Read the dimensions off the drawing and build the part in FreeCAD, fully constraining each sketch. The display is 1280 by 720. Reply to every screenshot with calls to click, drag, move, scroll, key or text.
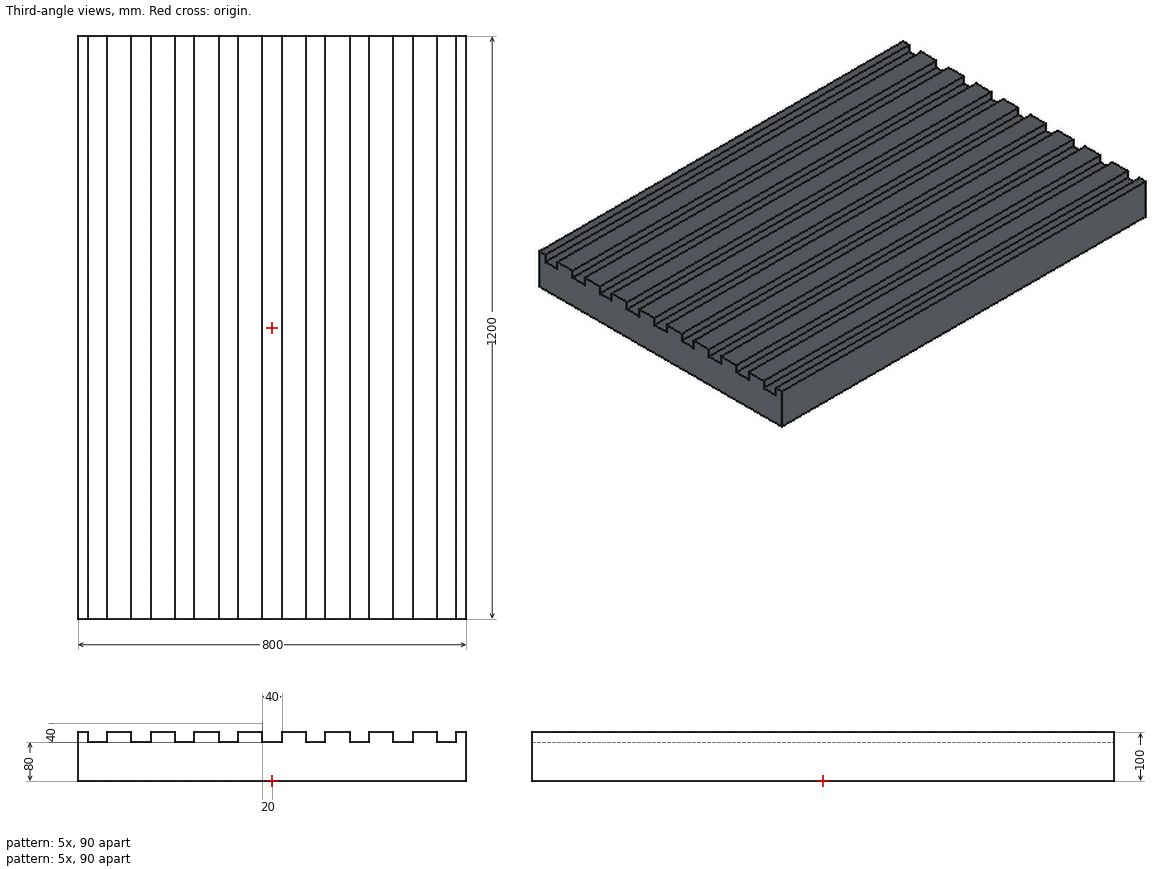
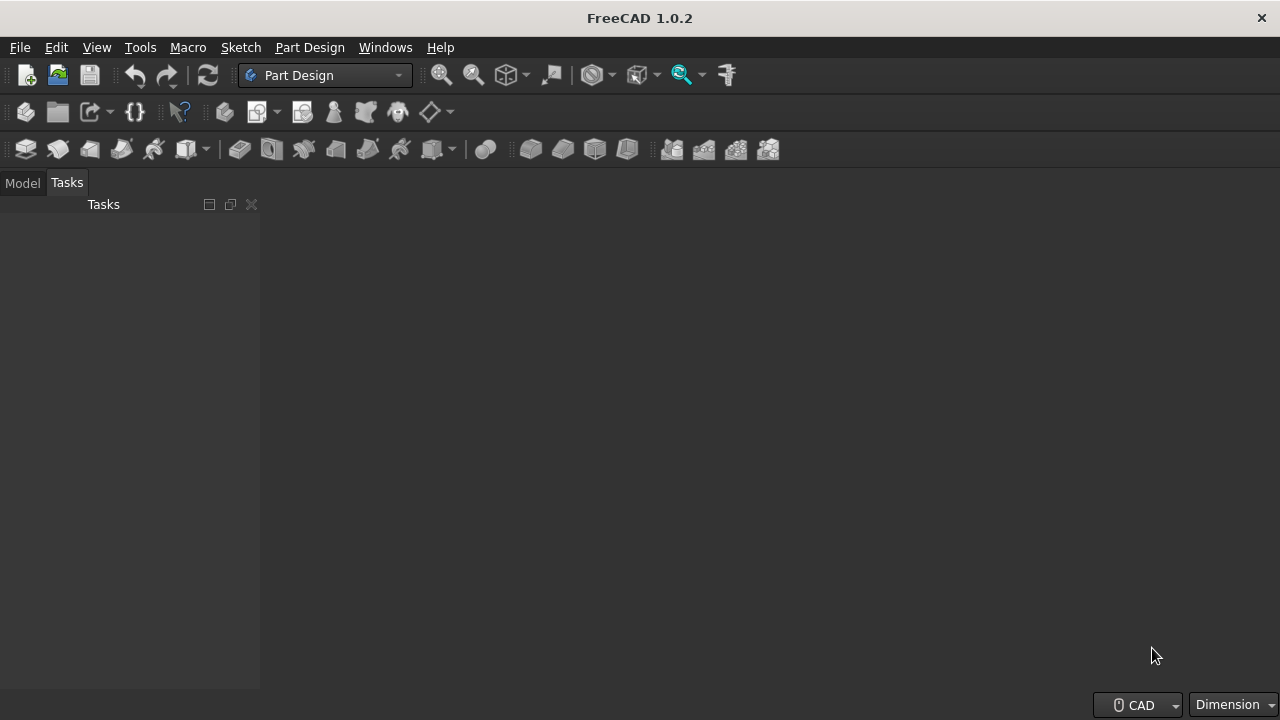
key(ctrl+n)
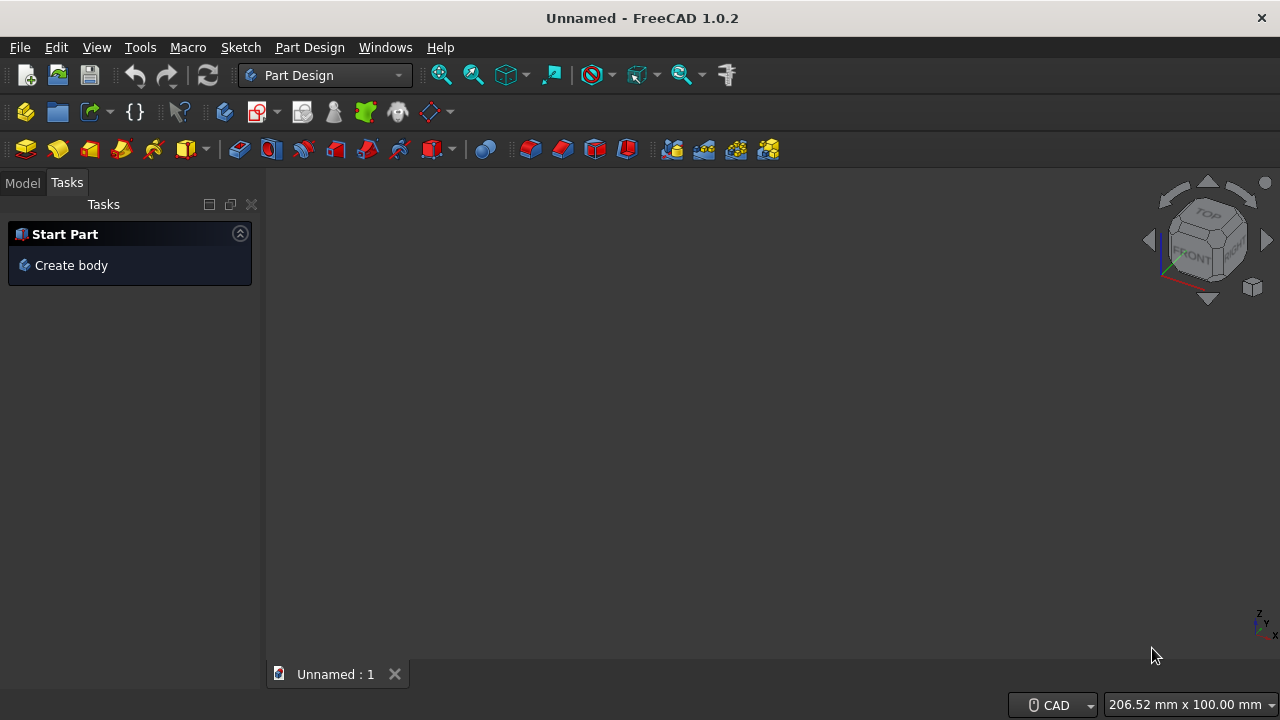
click(258, 112)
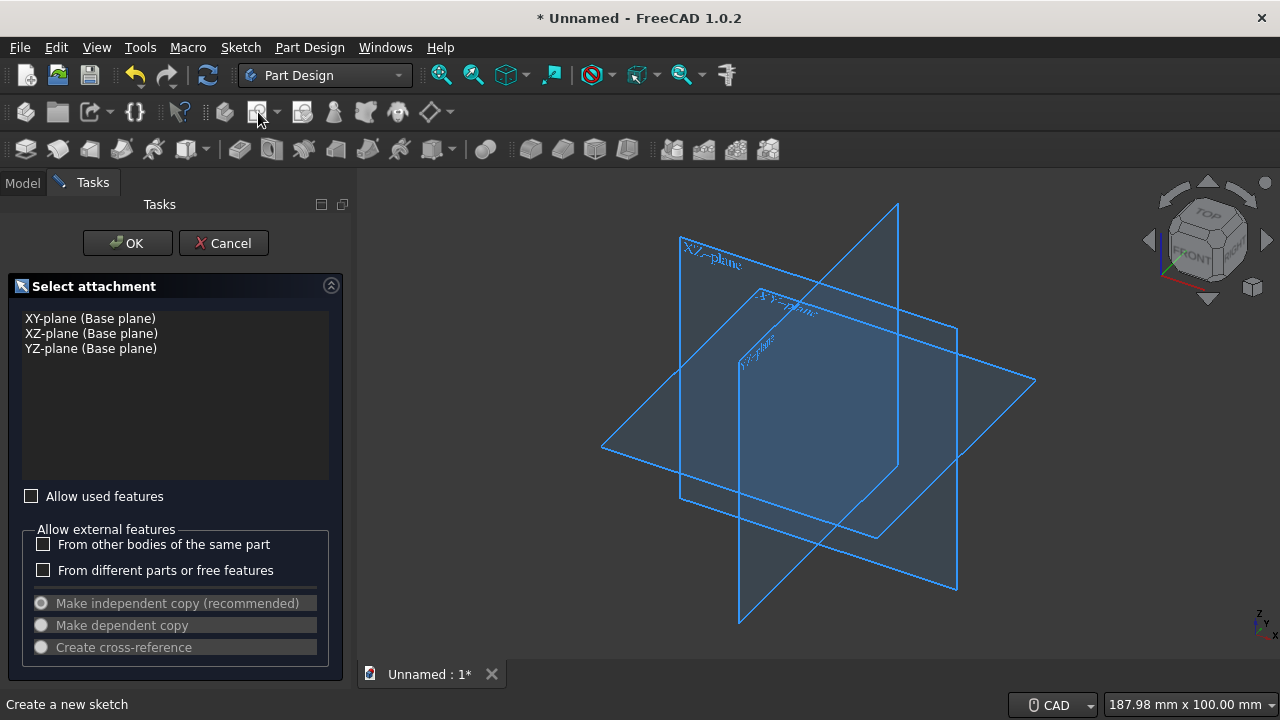
click(82, 318)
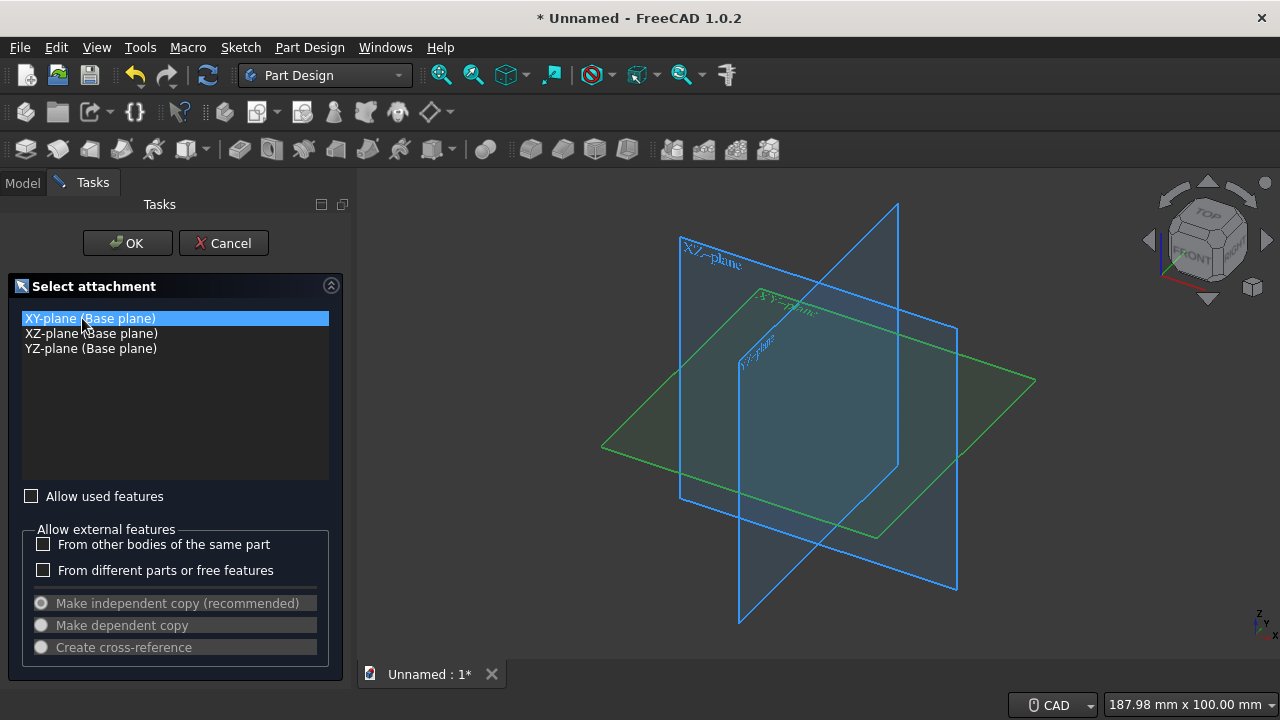
click(128, 243)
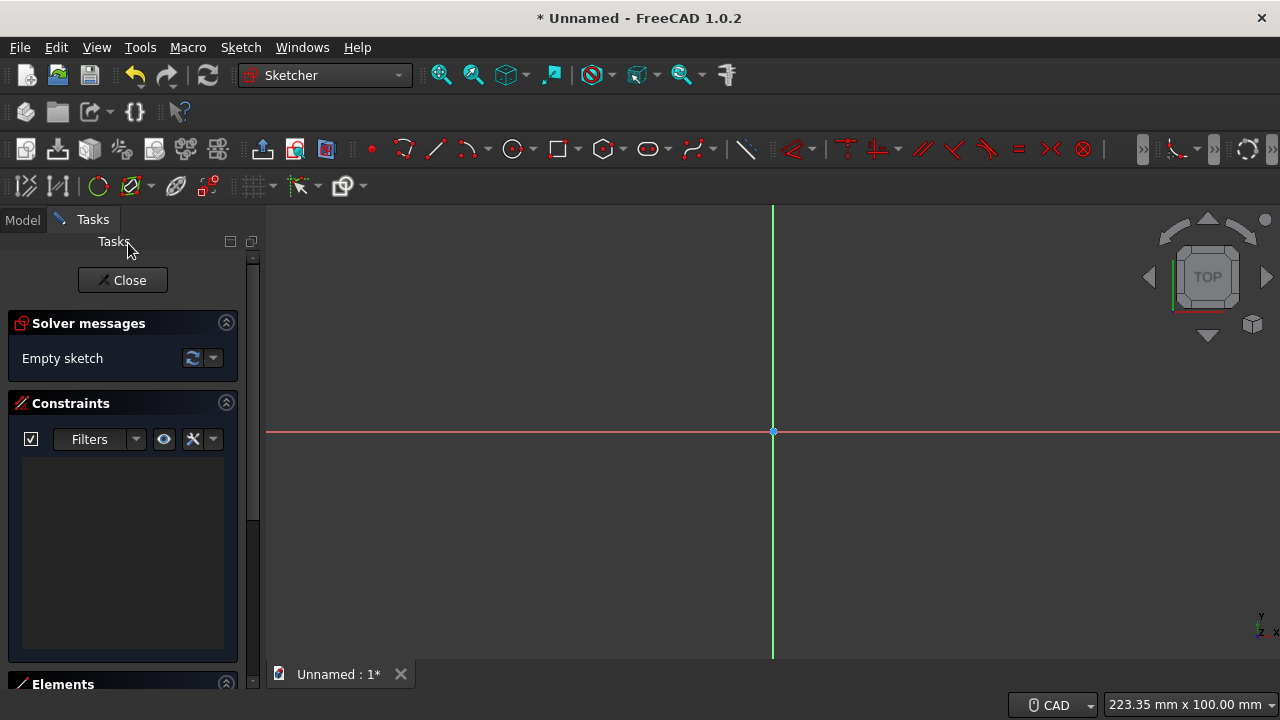
scroll(701, 432, down, 15)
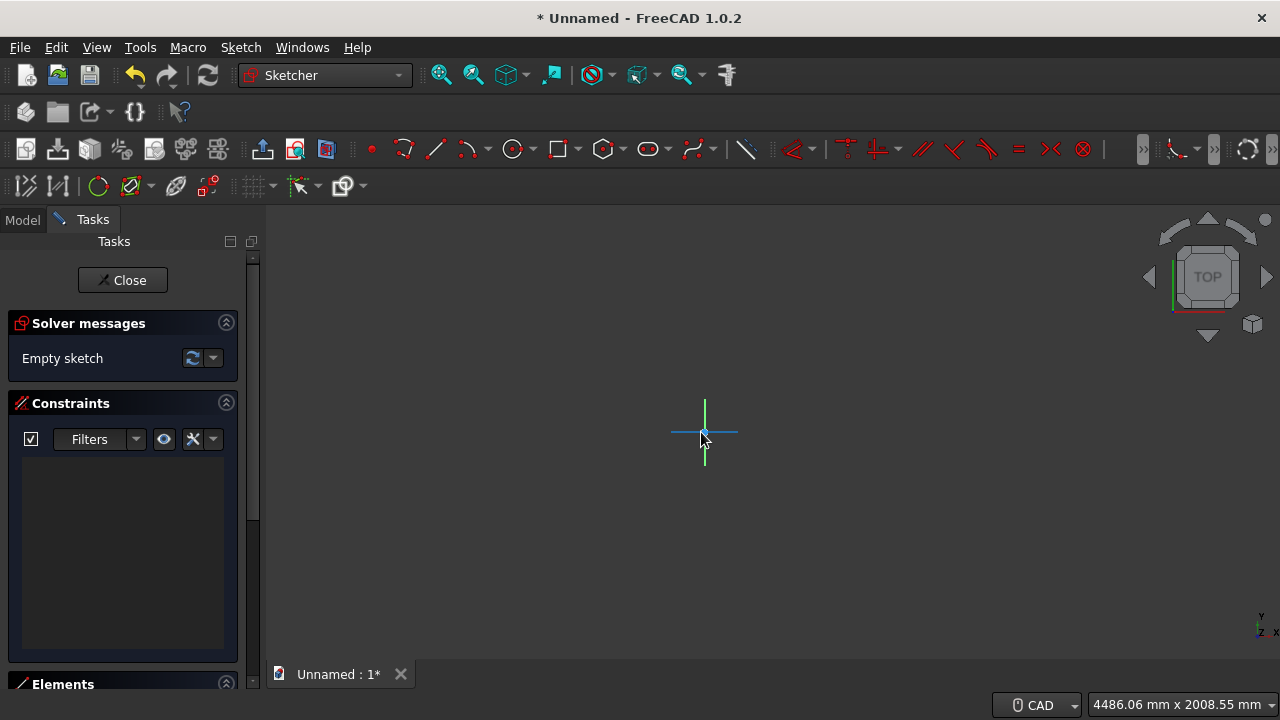
key(g)
key(v)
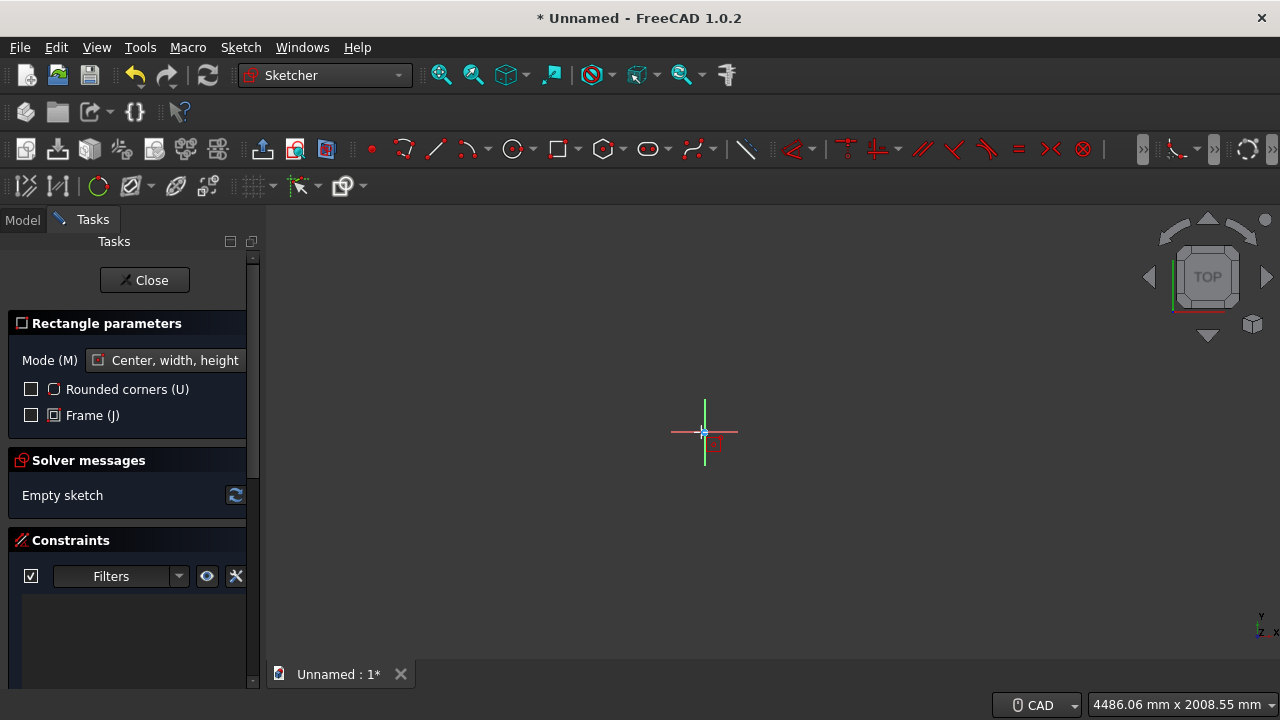
click(705, 432)
click(795, 297)
key(Escape)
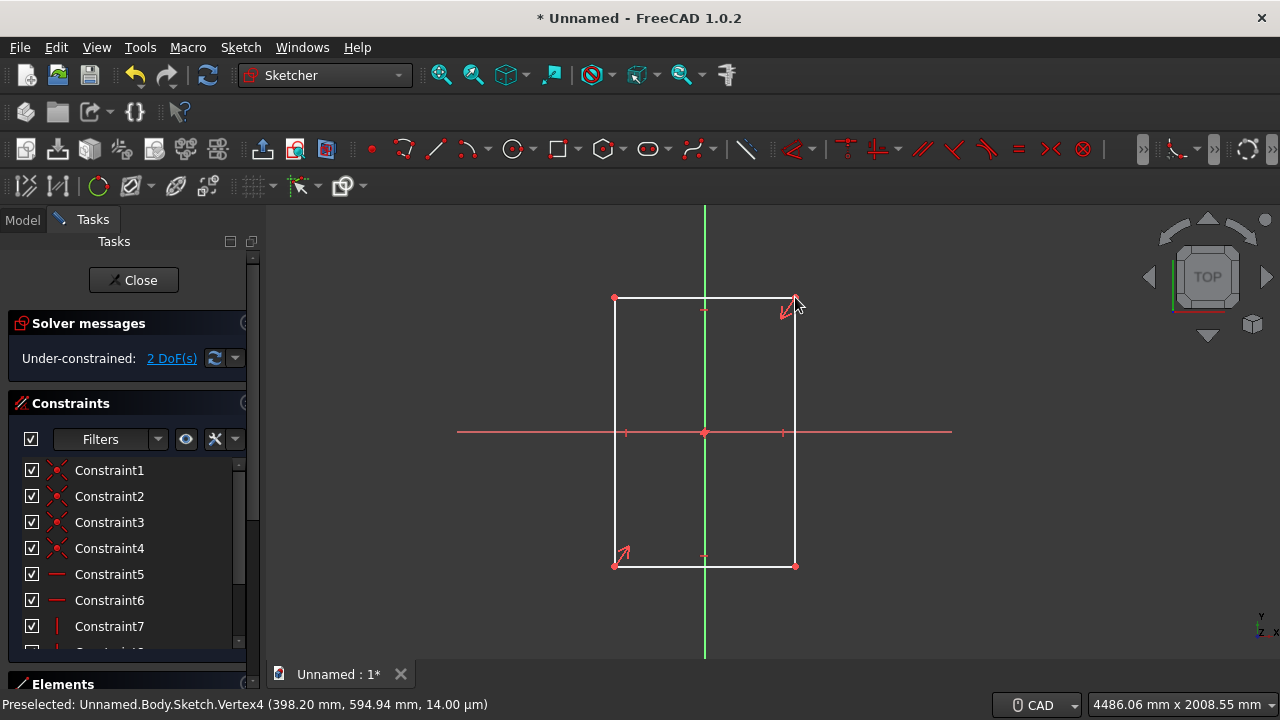
click(792, 150)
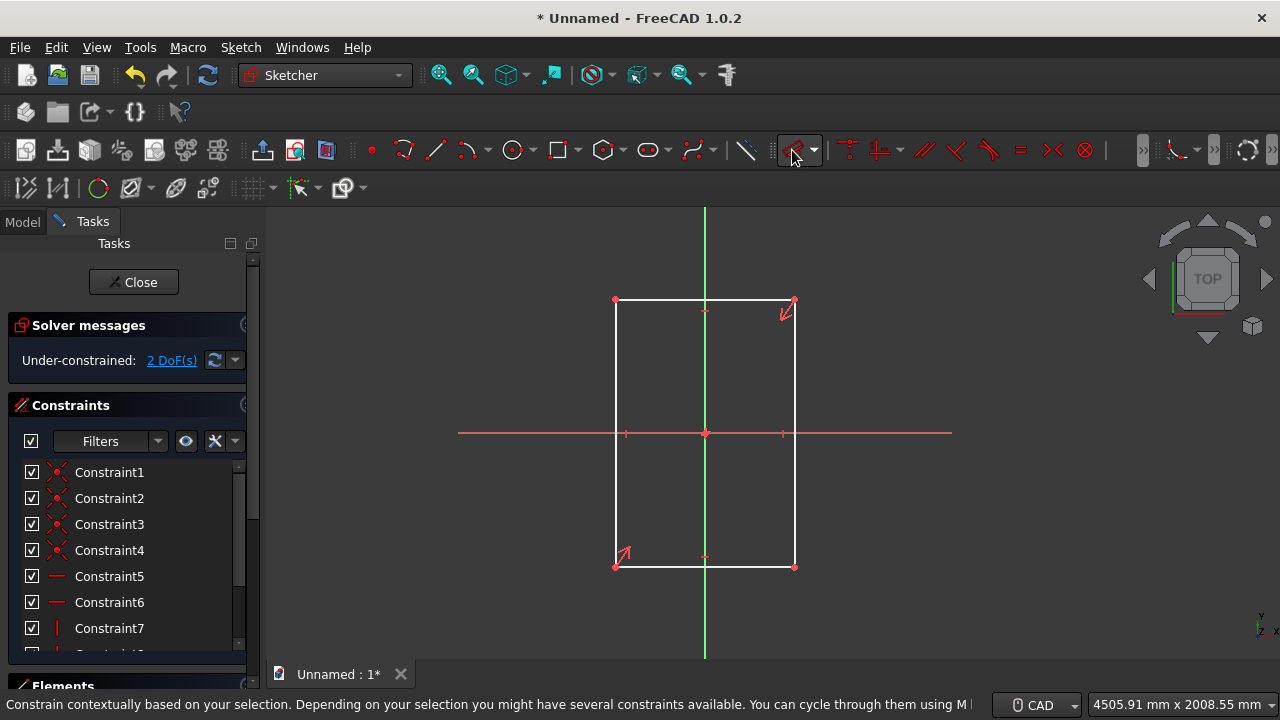
click(669, 567)
click(664, 601)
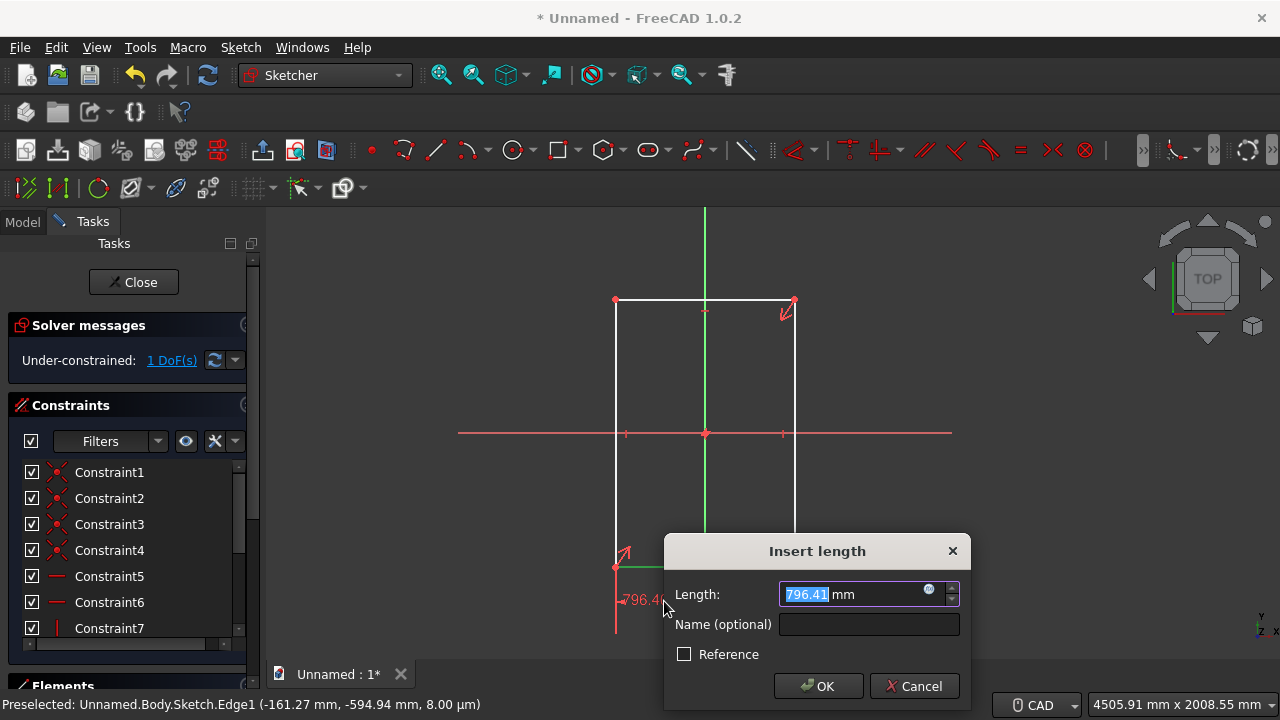
text(800)
key(Return)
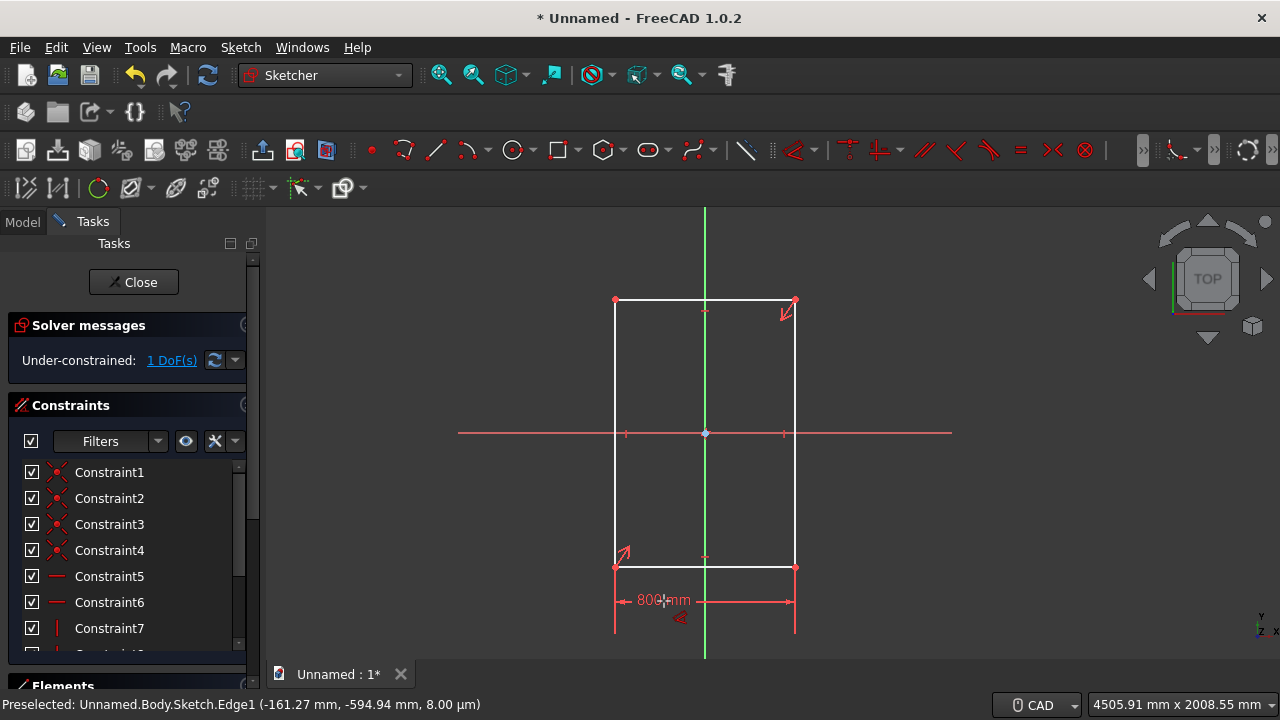
click(795, 487)
click(829, 372)